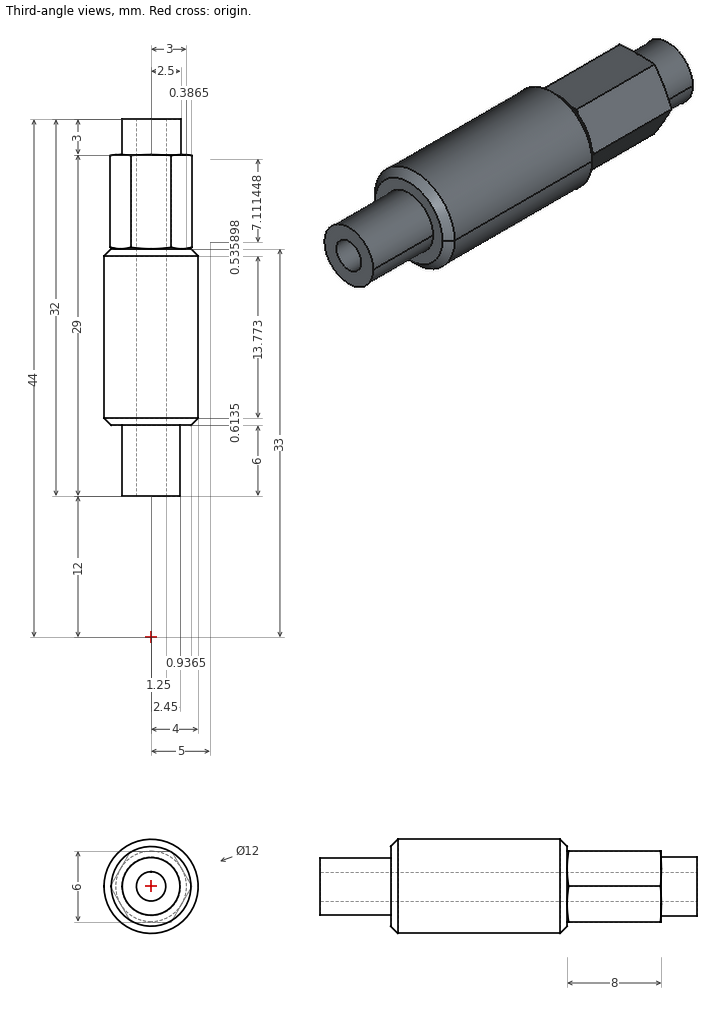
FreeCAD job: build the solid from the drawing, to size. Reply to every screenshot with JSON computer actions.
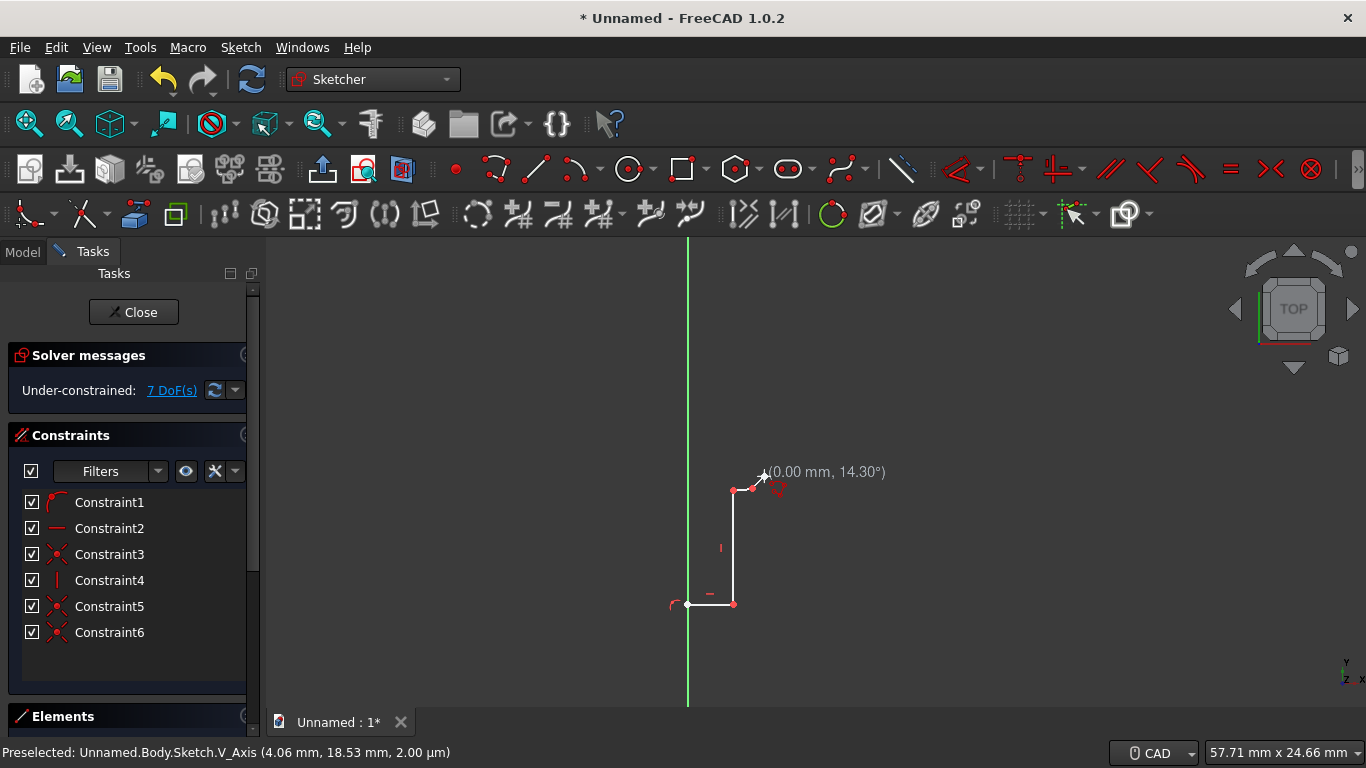
{"action": "scroll", "coordinate": [755, 490], "scroll_direction": "down", "scroll_amount": 5}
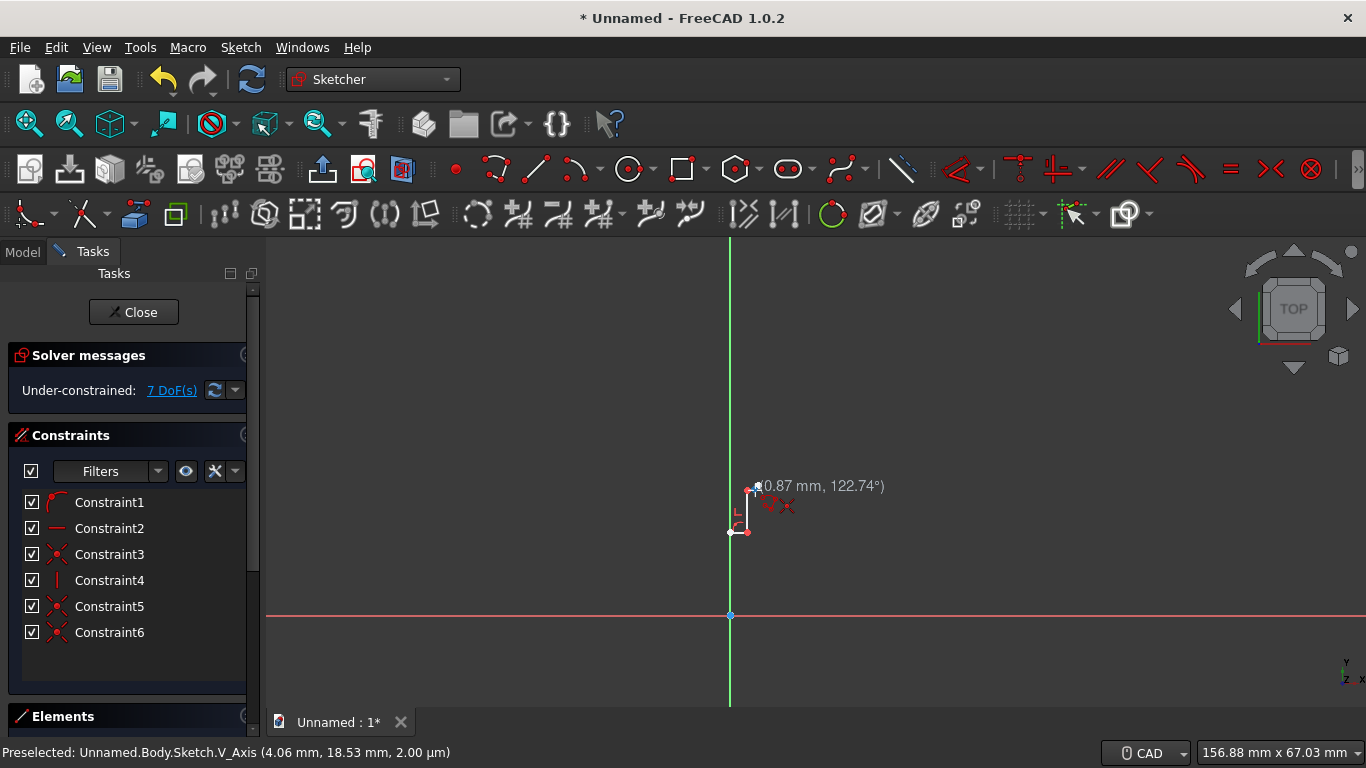
{"action": "left_click", "coordinate": [759, 389]}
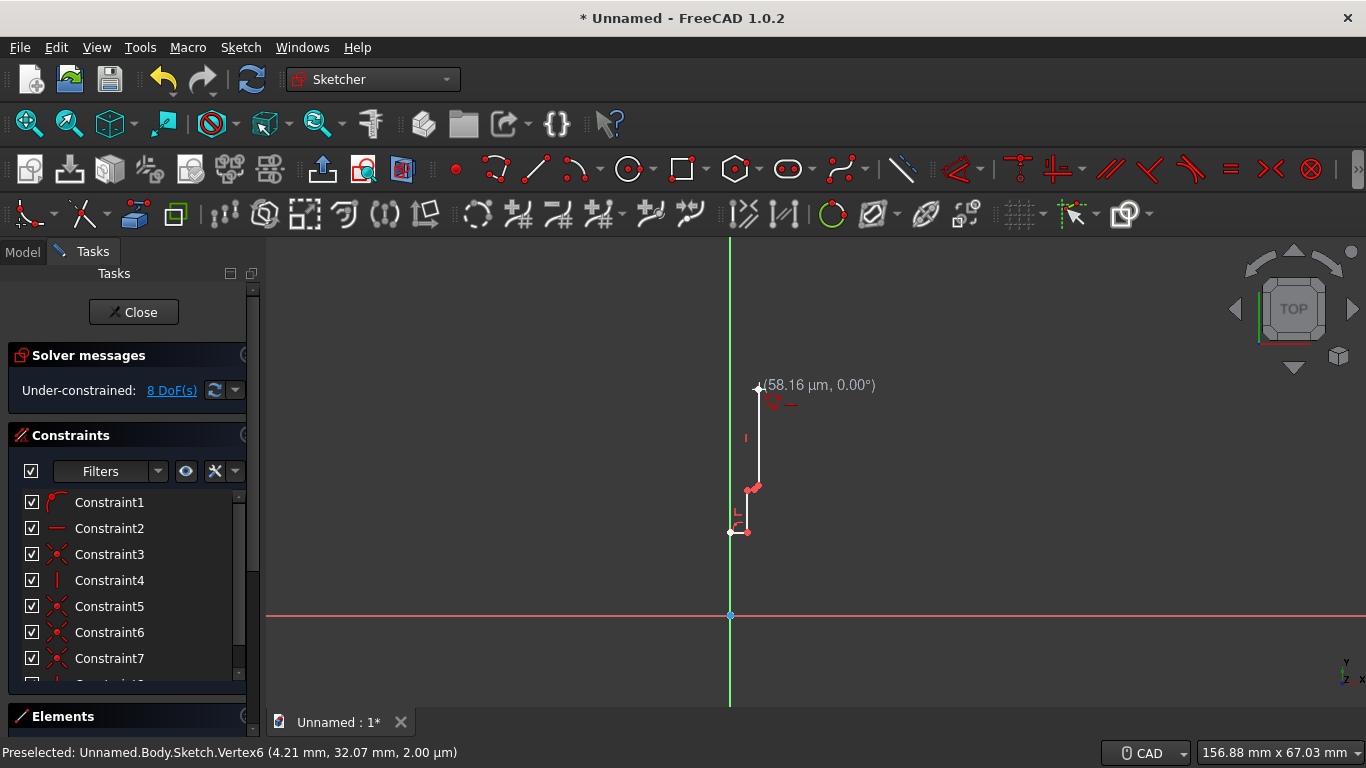
{"action": "scroll", "coordinate": [754, 384], "scroll_direction": "up", "scroll_amount": 5}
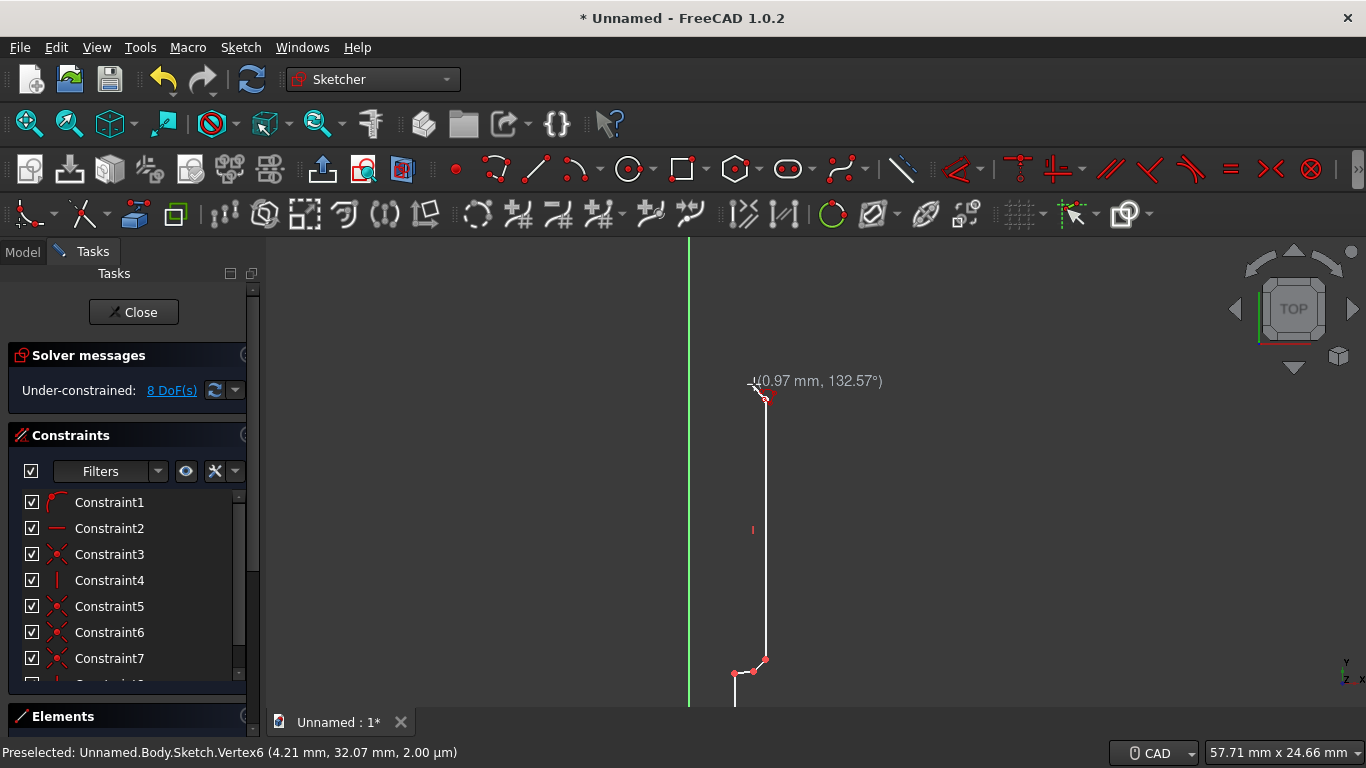
{"action": "left_click", "coordinate": [754, 385]}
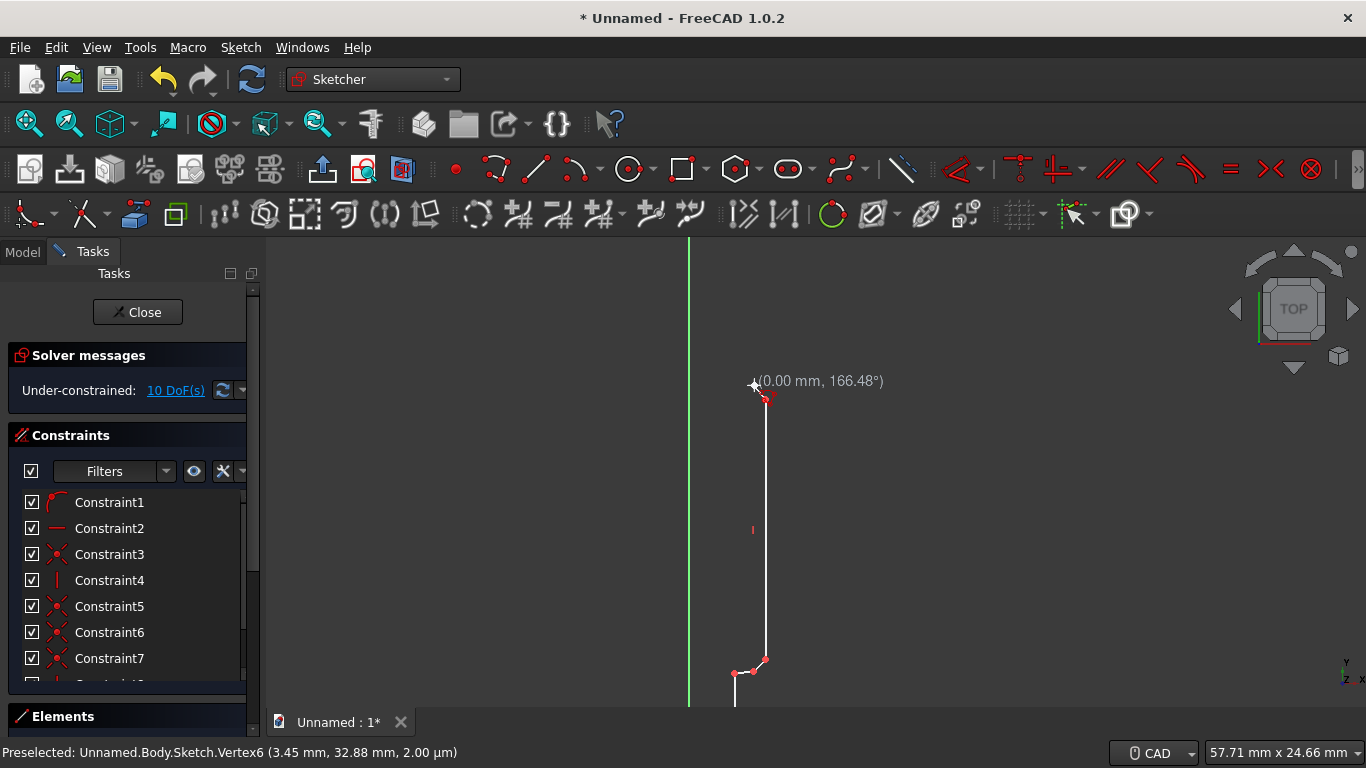
{"action": "scroll", "coordinate": [747, 385], "scroll_direction": "up", "scroll_amount": 4}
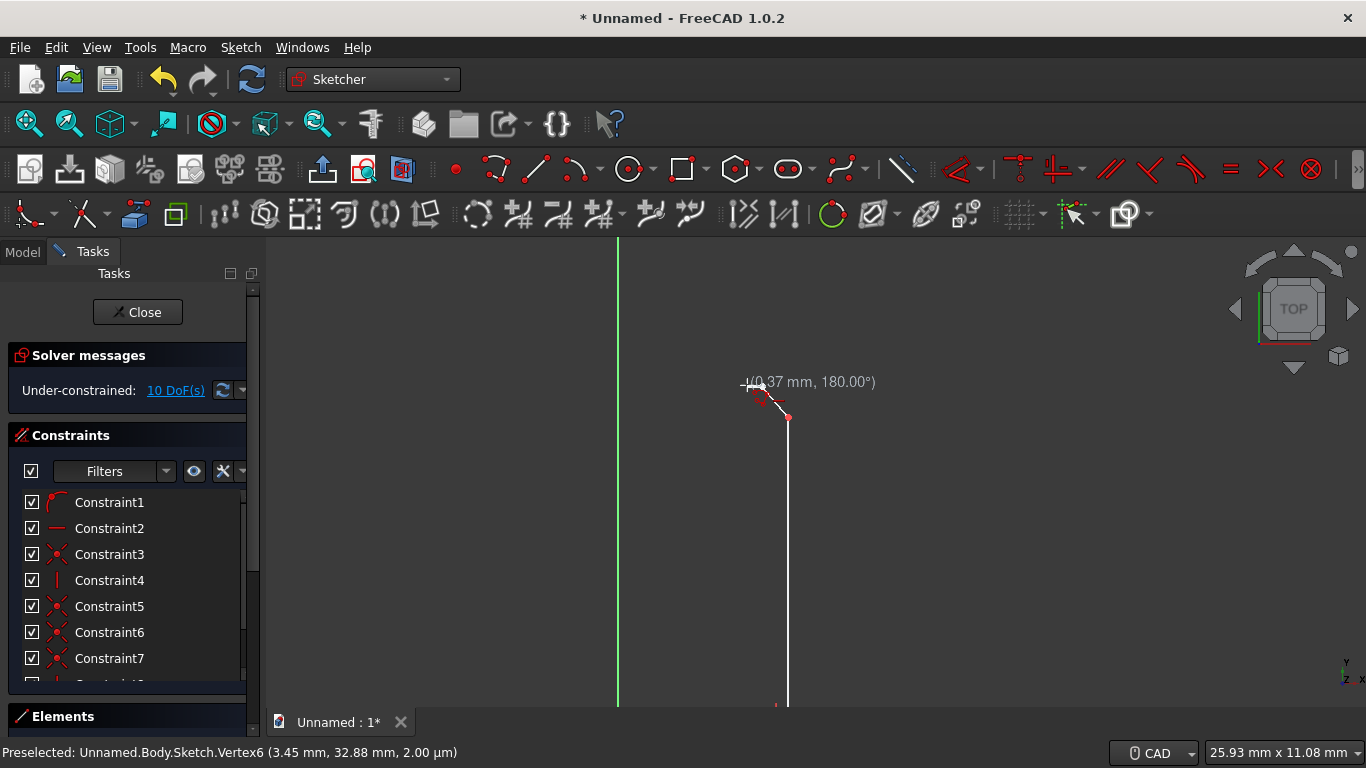
{"action": "left_click", "coordinate": [745, 385]}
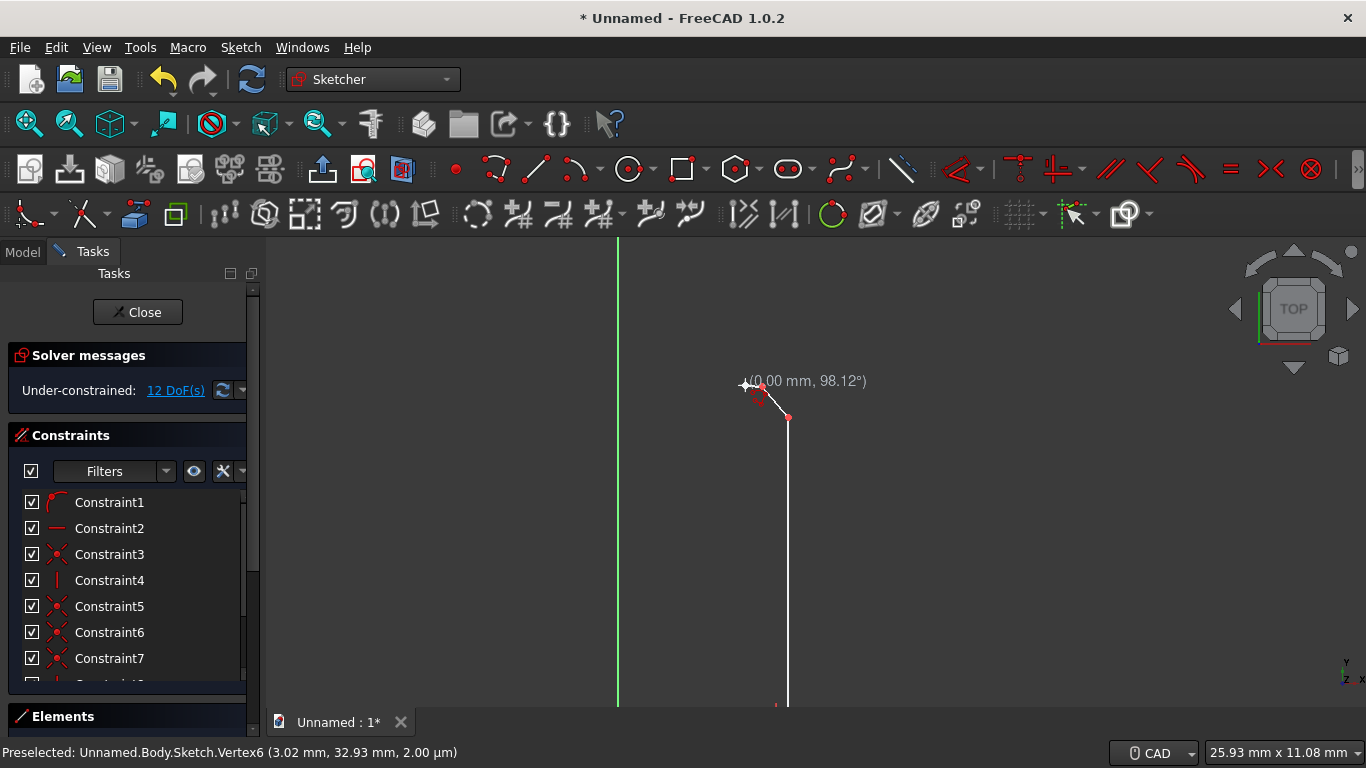
{"action": "scroll", "coordinate": [752, 384], "scroll_direction": "down", "scroll_amount": 9}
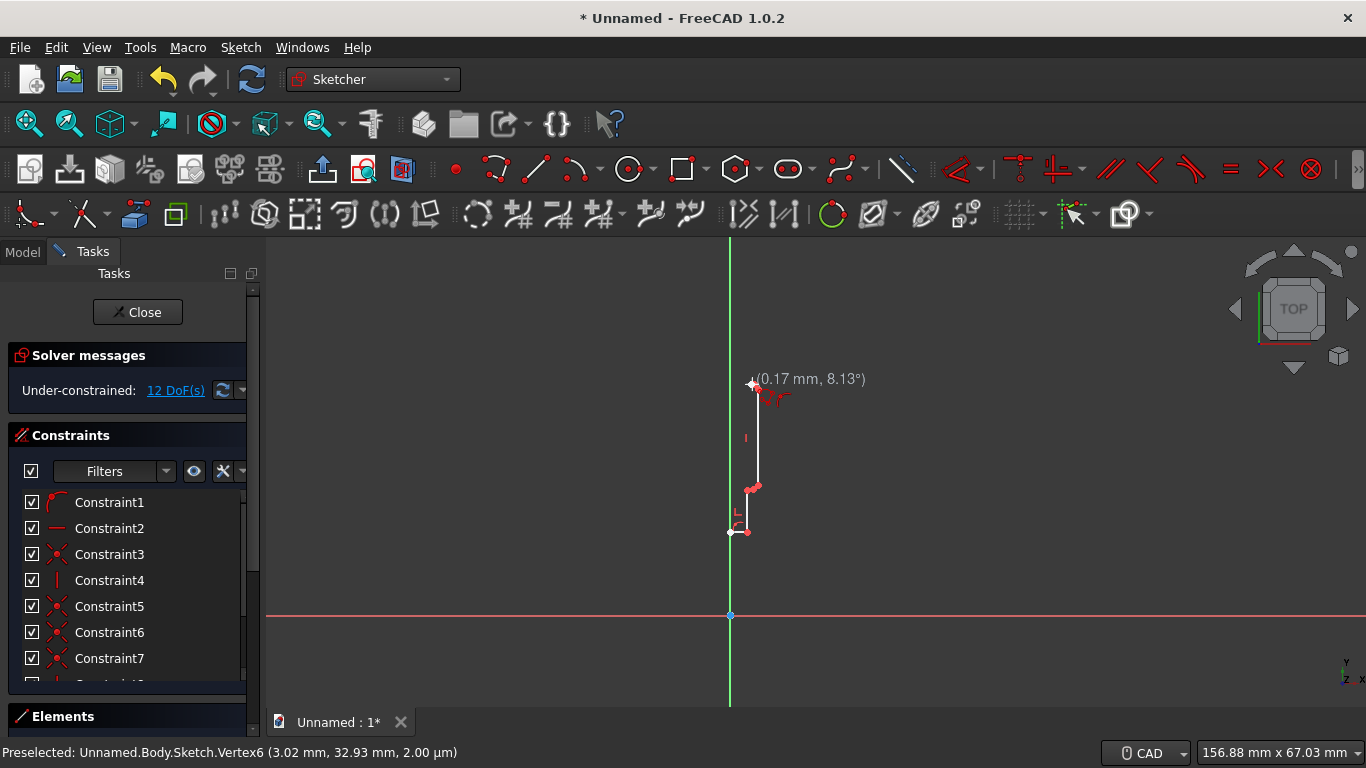
{"action": "scroll", "coordinate": [765, 381], "scroll_direction": "up", "scroll_amount": 2}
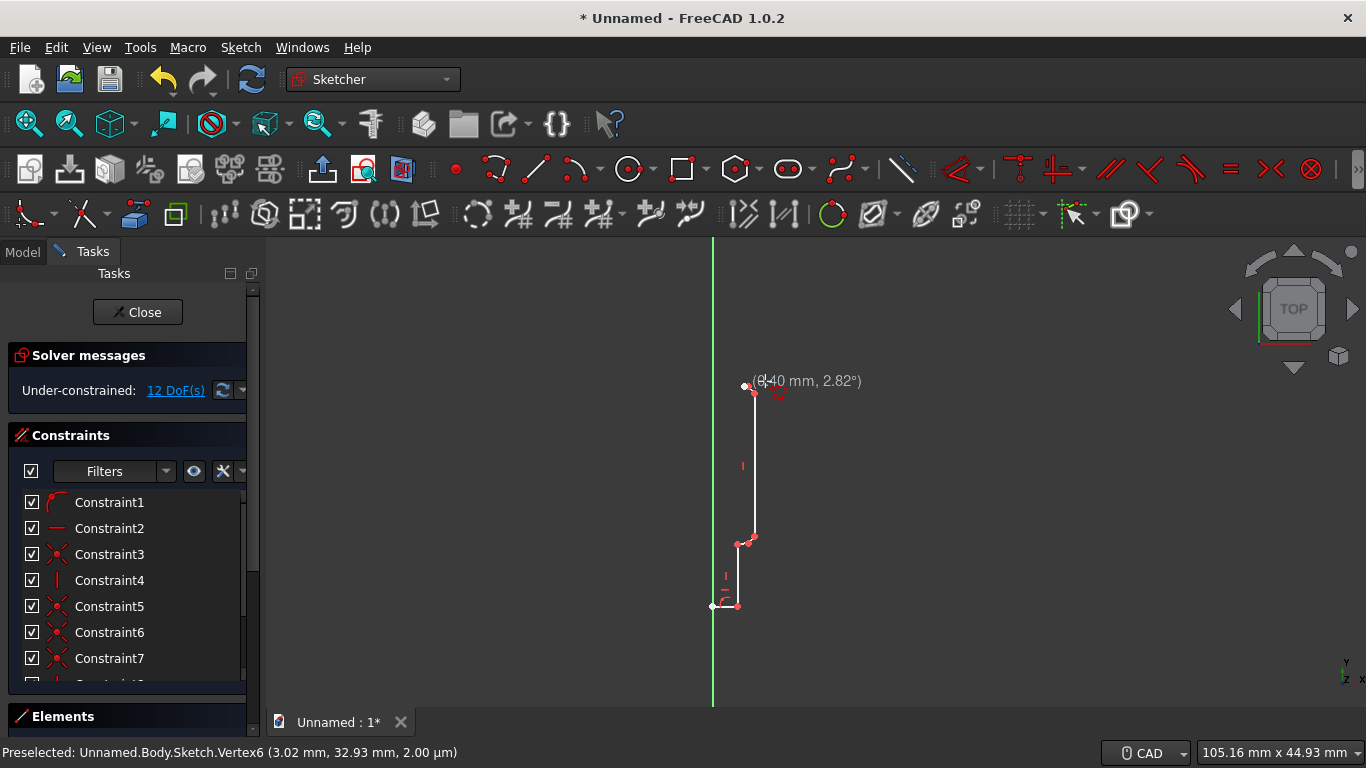
{"action": "left_click", "coordinate": [765, 380]}
{"action": "left_click", "coordinate": [765, 306]}
{"action": "left_click", "coordinate": [744, 302]}
{"action": "left_click", "coordinate": [722, 302]}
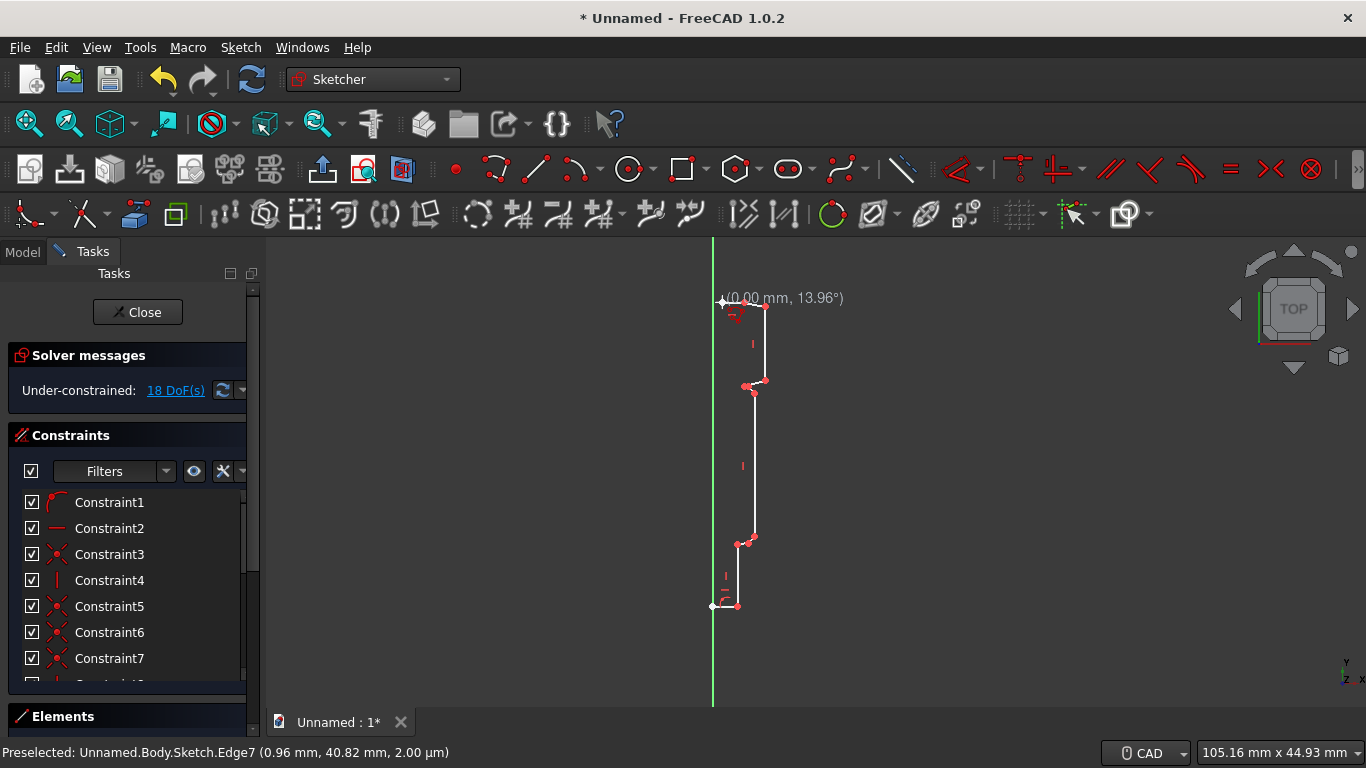
{"action": "scroll", "coordinate": [713, 605], "scroll_direction": "up", "scroll_amount": 2}